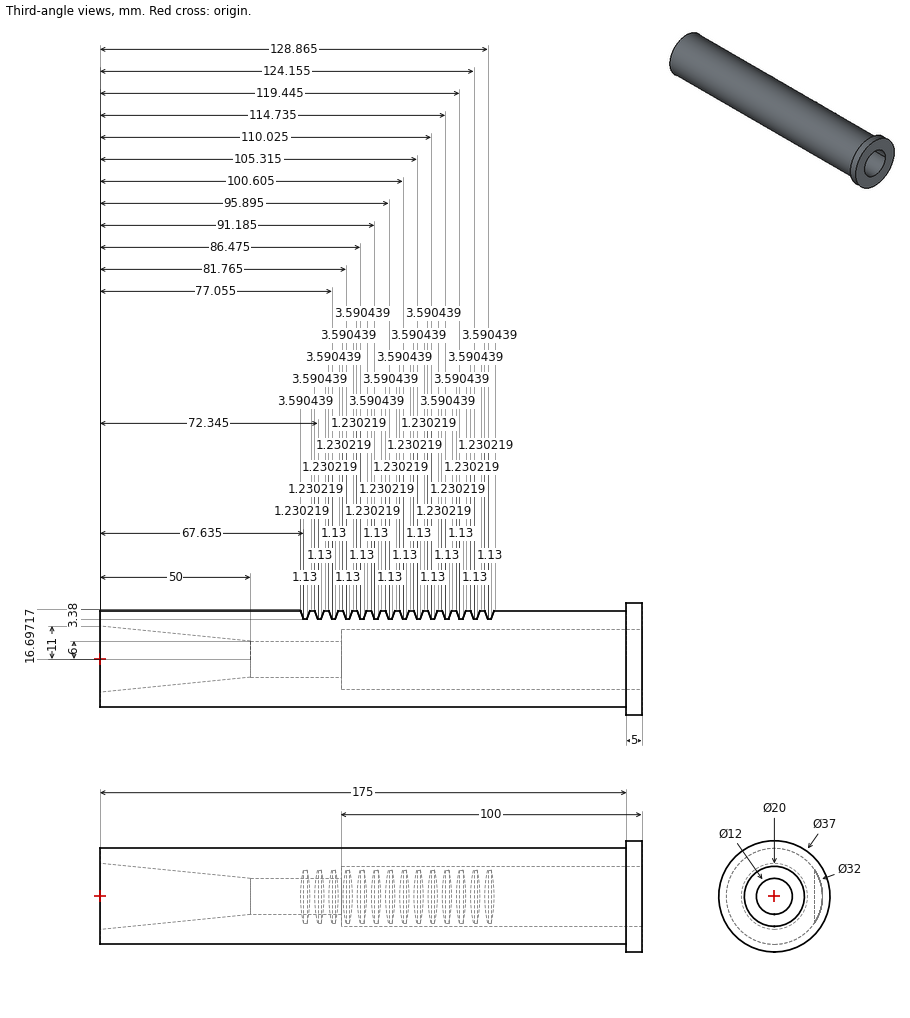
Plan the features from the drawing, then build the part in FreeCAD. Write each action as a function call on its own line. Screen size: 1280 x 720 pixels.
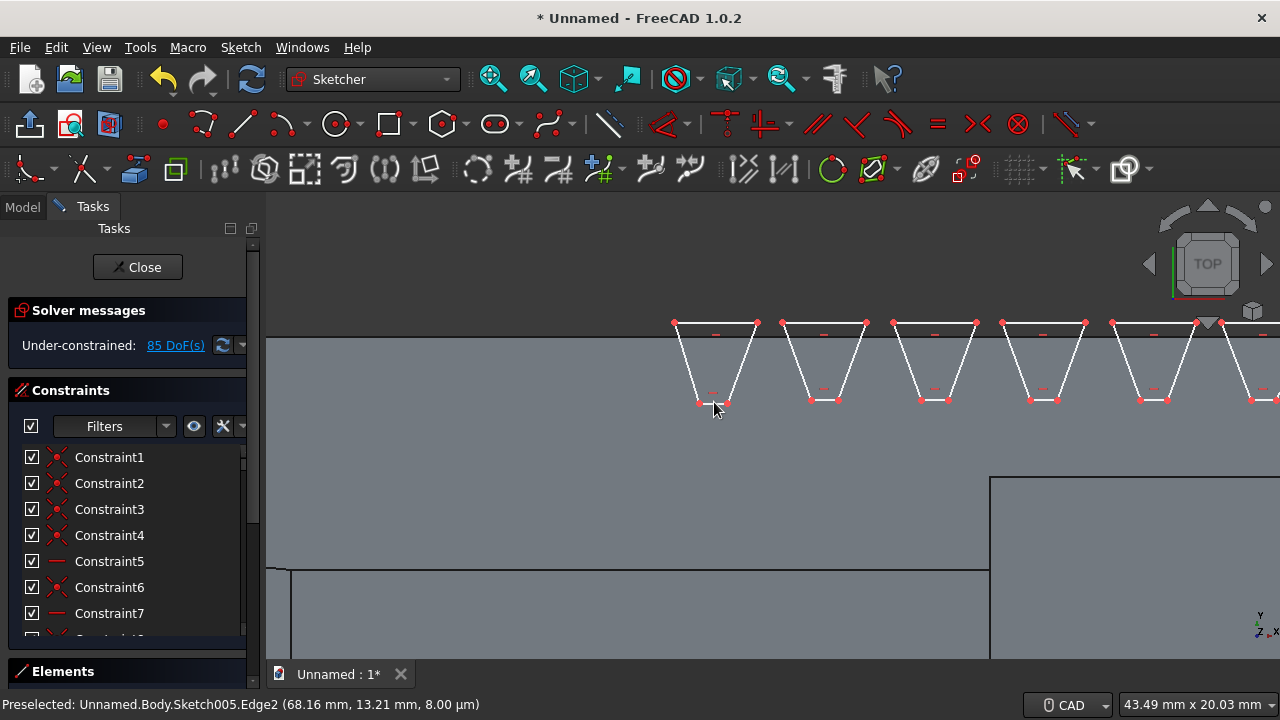
scroll(717, 403, down, 8)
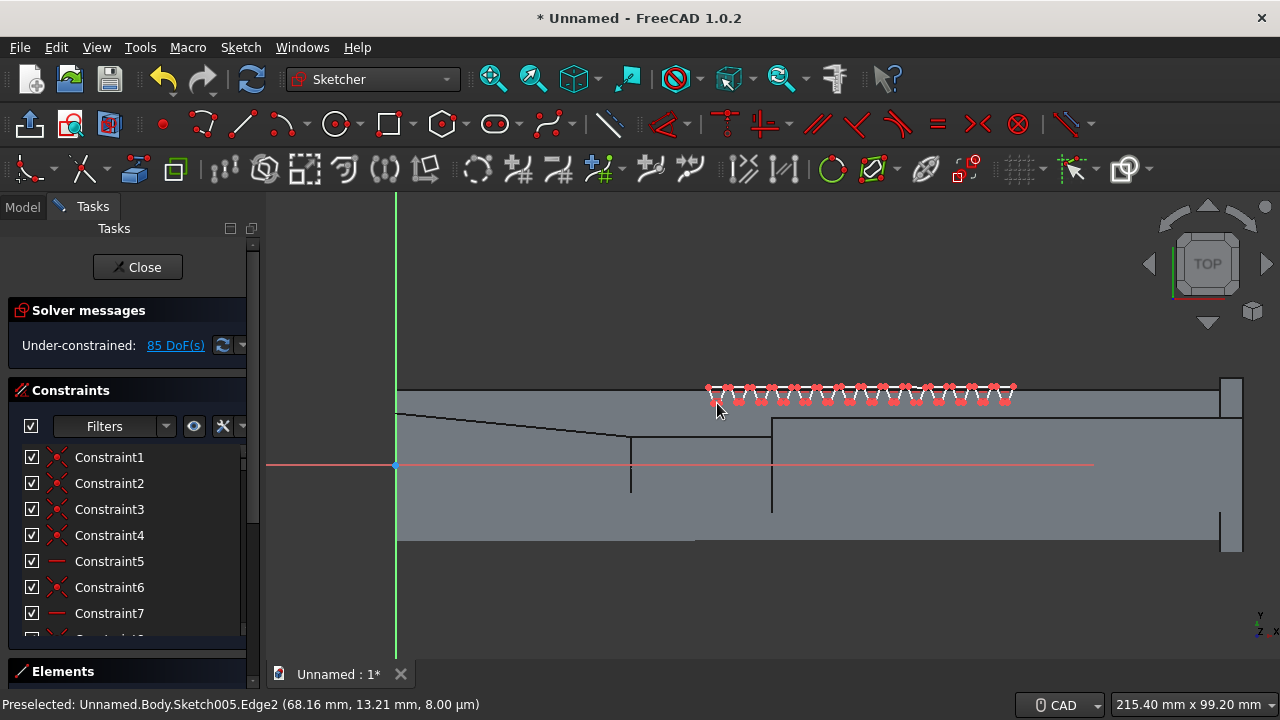
scroll(920, 388, up, 6)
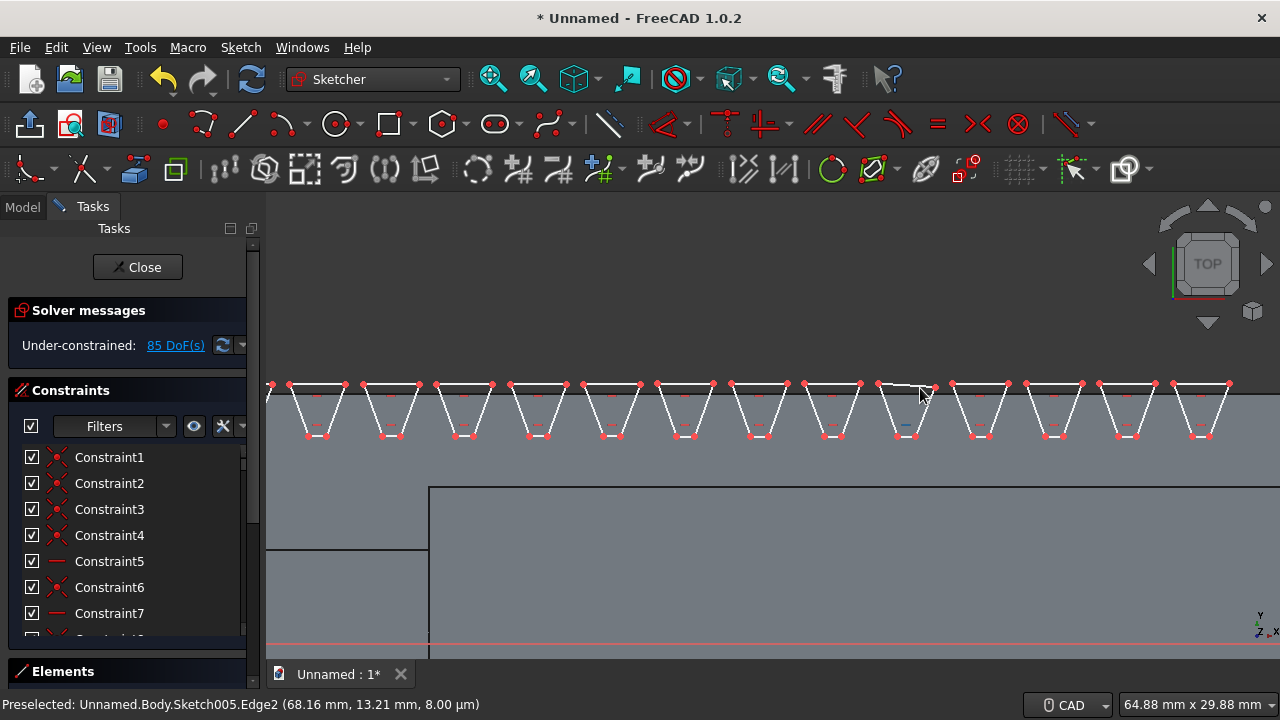
click(918, 386)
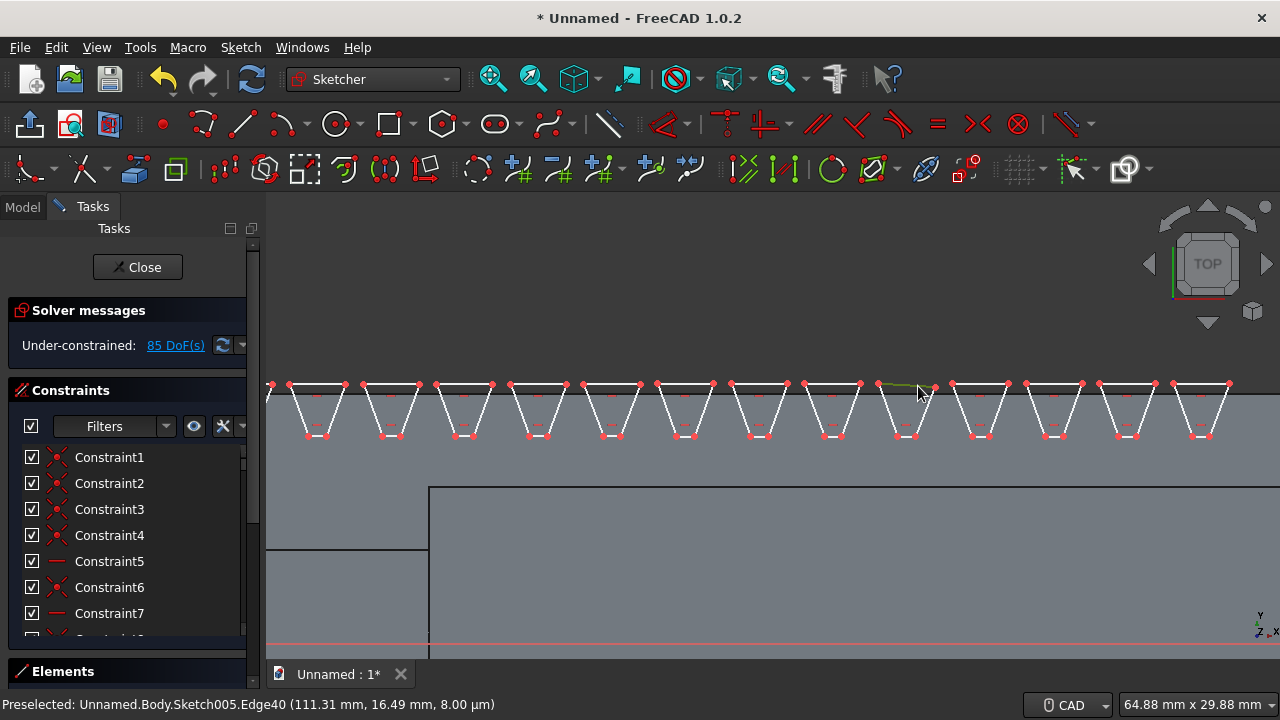
key(h)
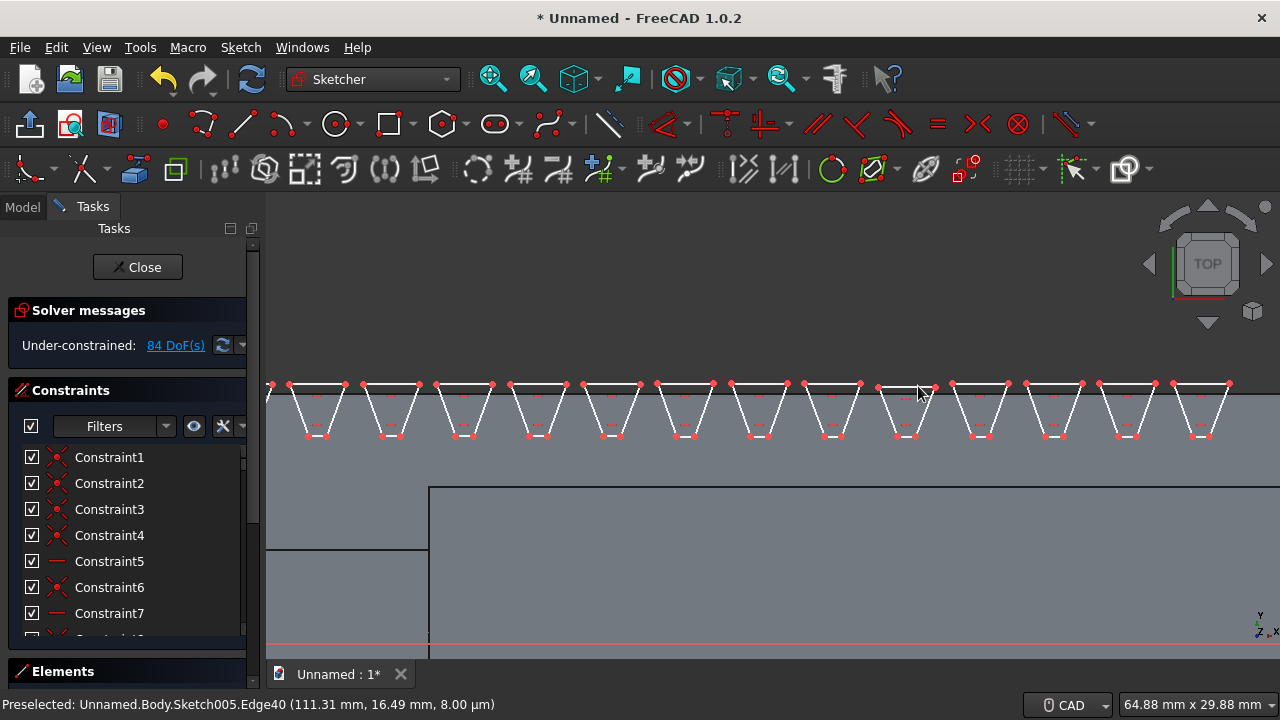
key(d)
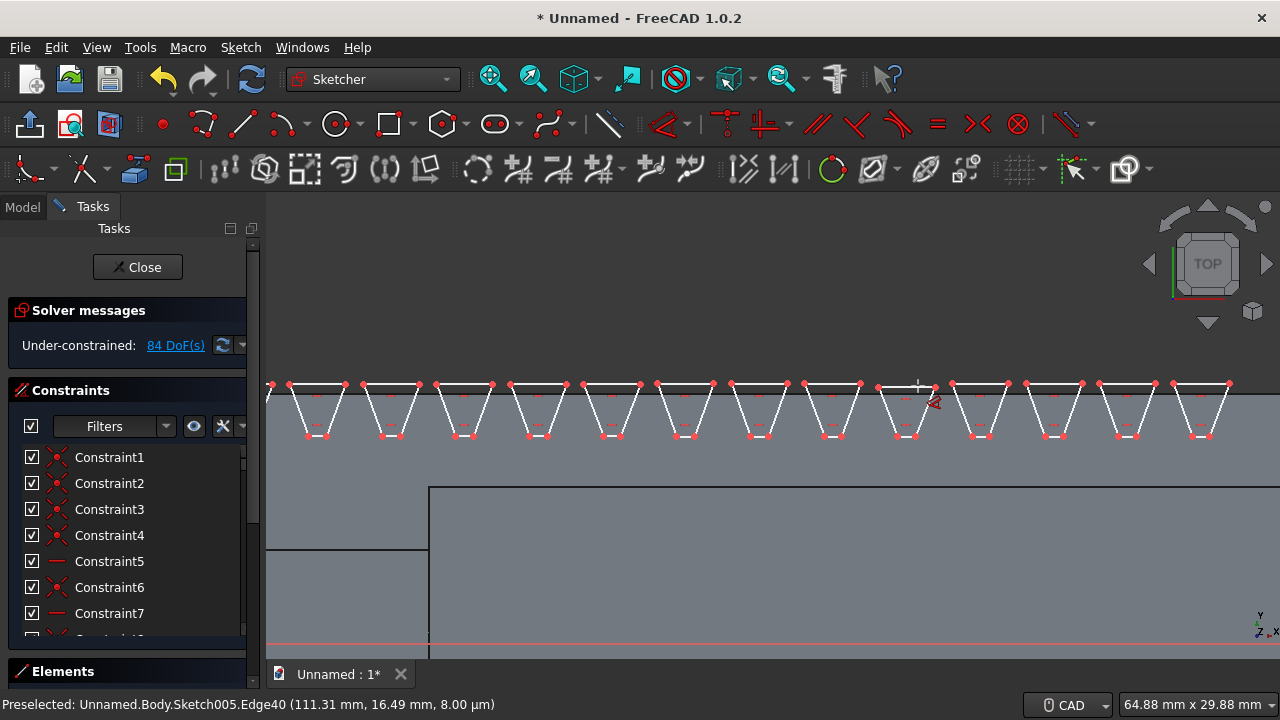
scroll(920, 388, down, 6)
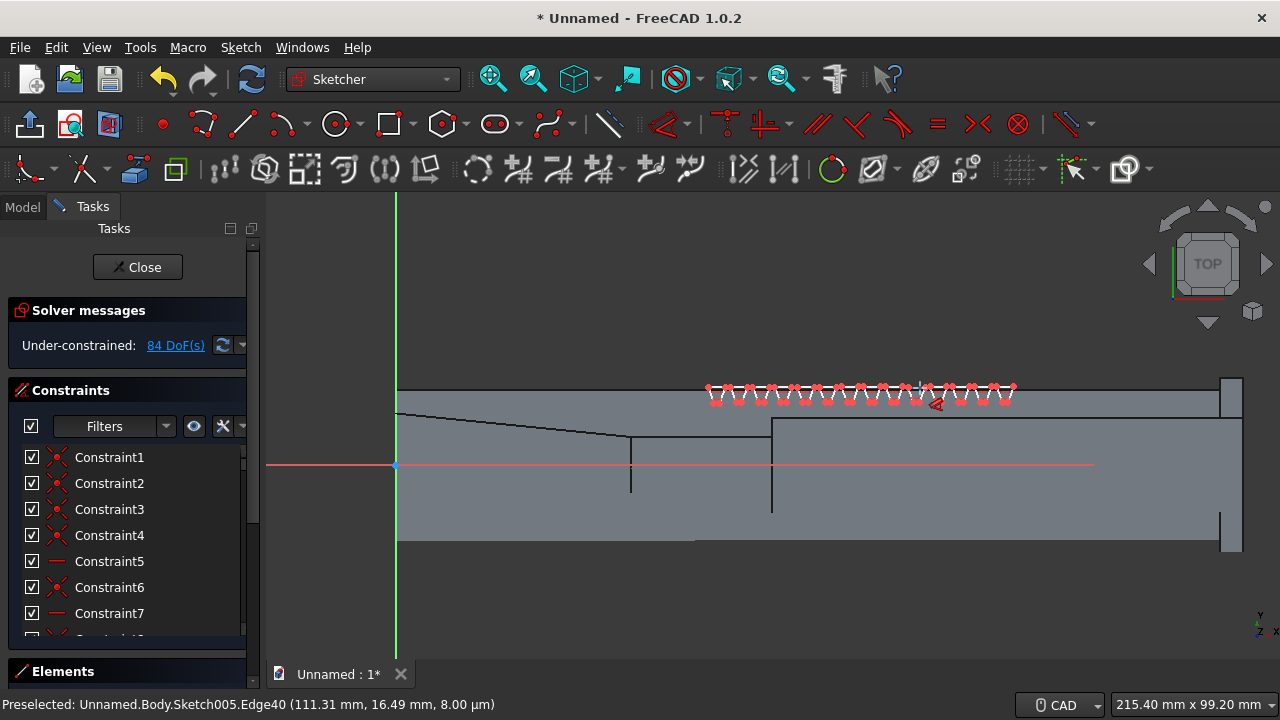
scroll(717, 404, up, 11)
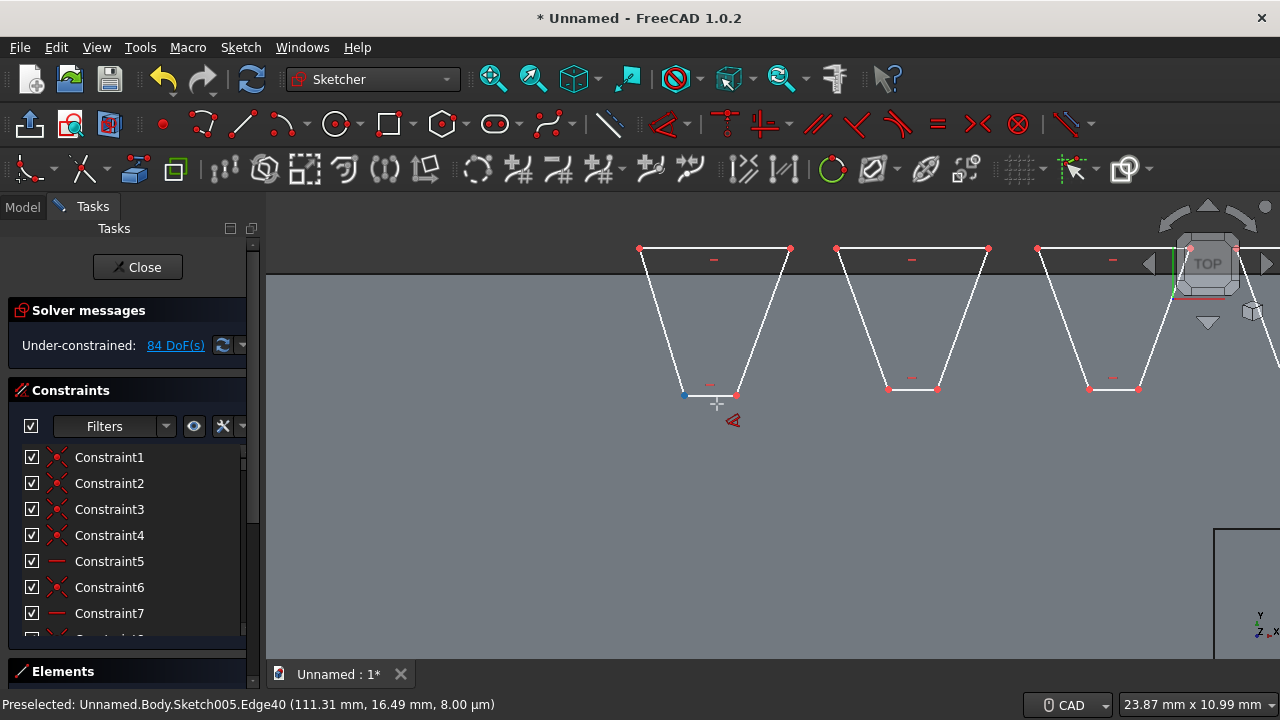
click(710, 396)
click(710, 362)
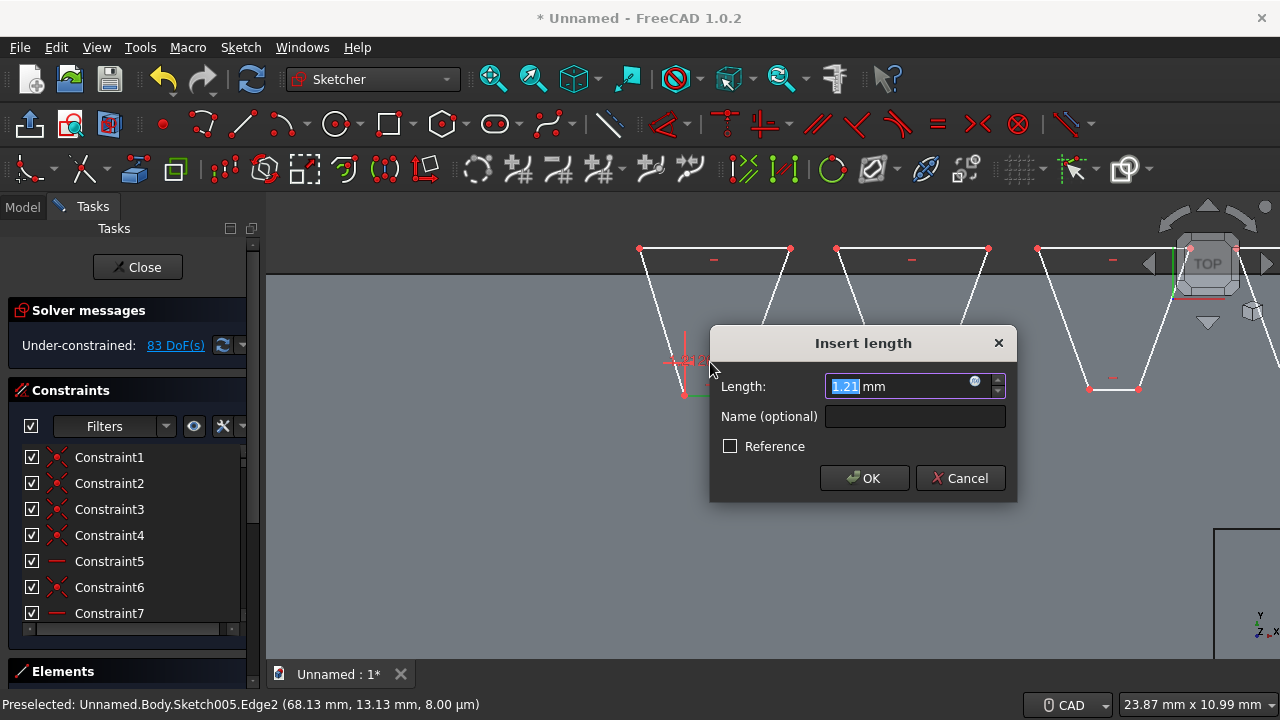
text(1.13)
key(Return)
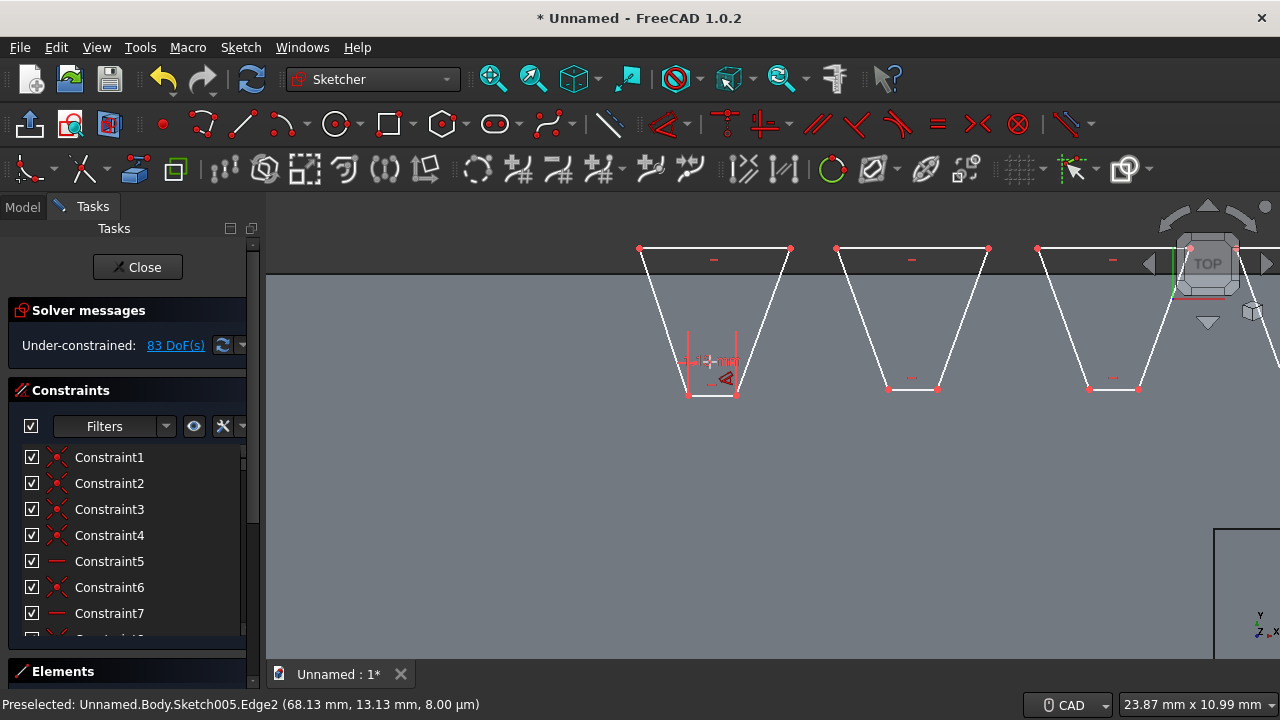
click(903, 390)
click(913, 356)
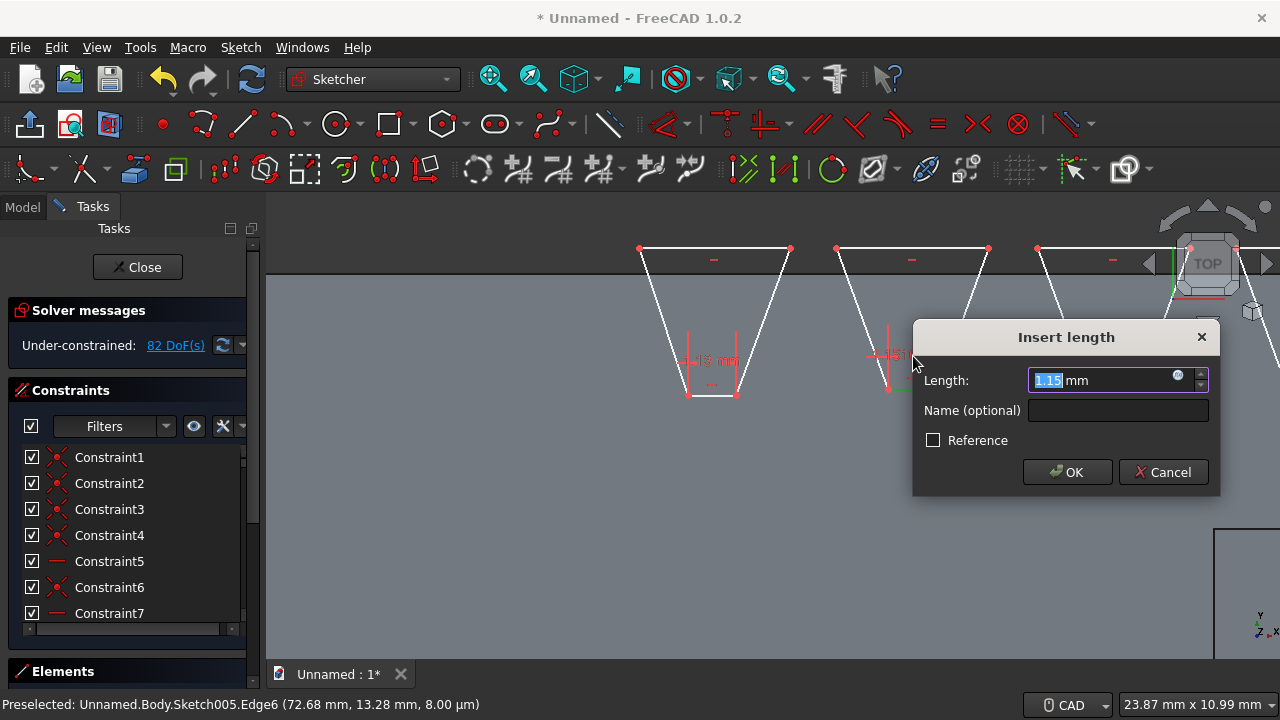
text(1.13)
key(Return)